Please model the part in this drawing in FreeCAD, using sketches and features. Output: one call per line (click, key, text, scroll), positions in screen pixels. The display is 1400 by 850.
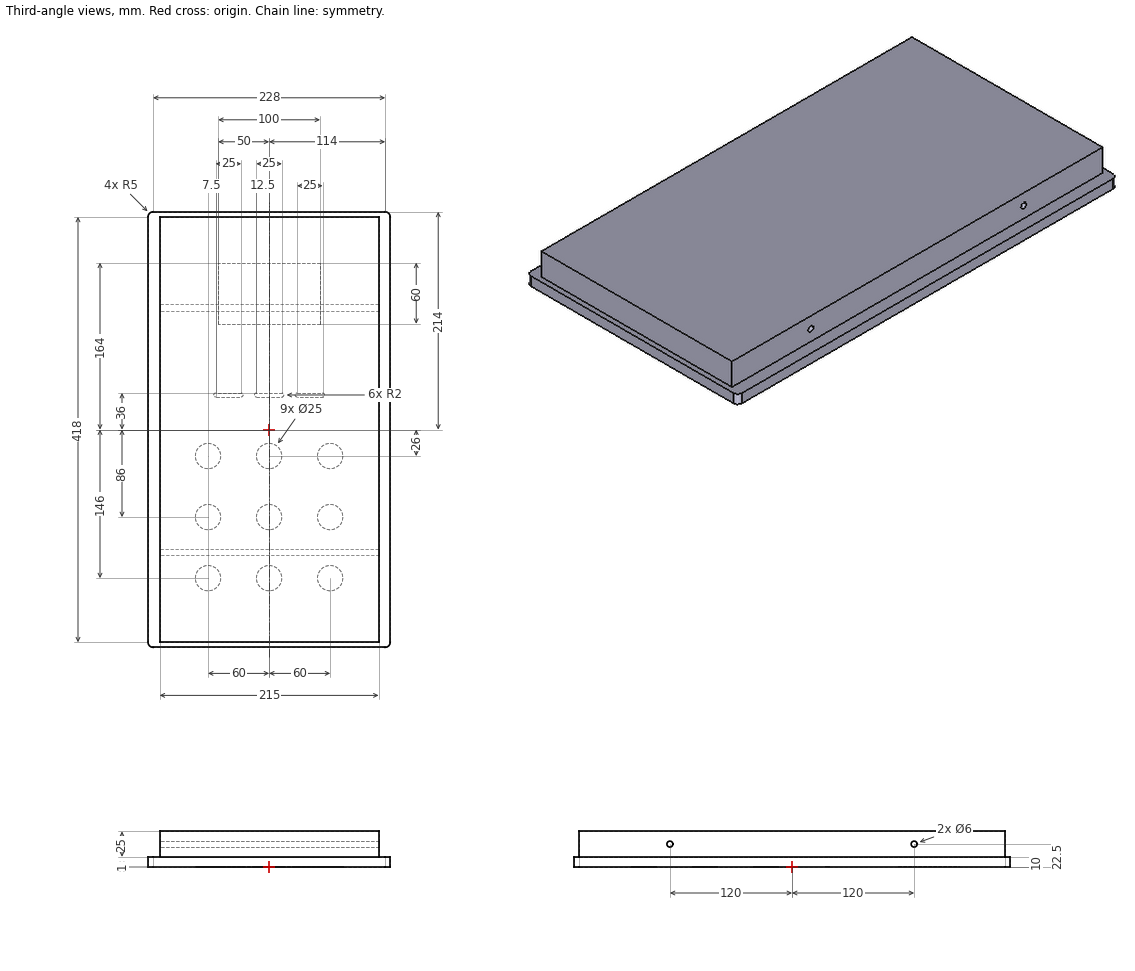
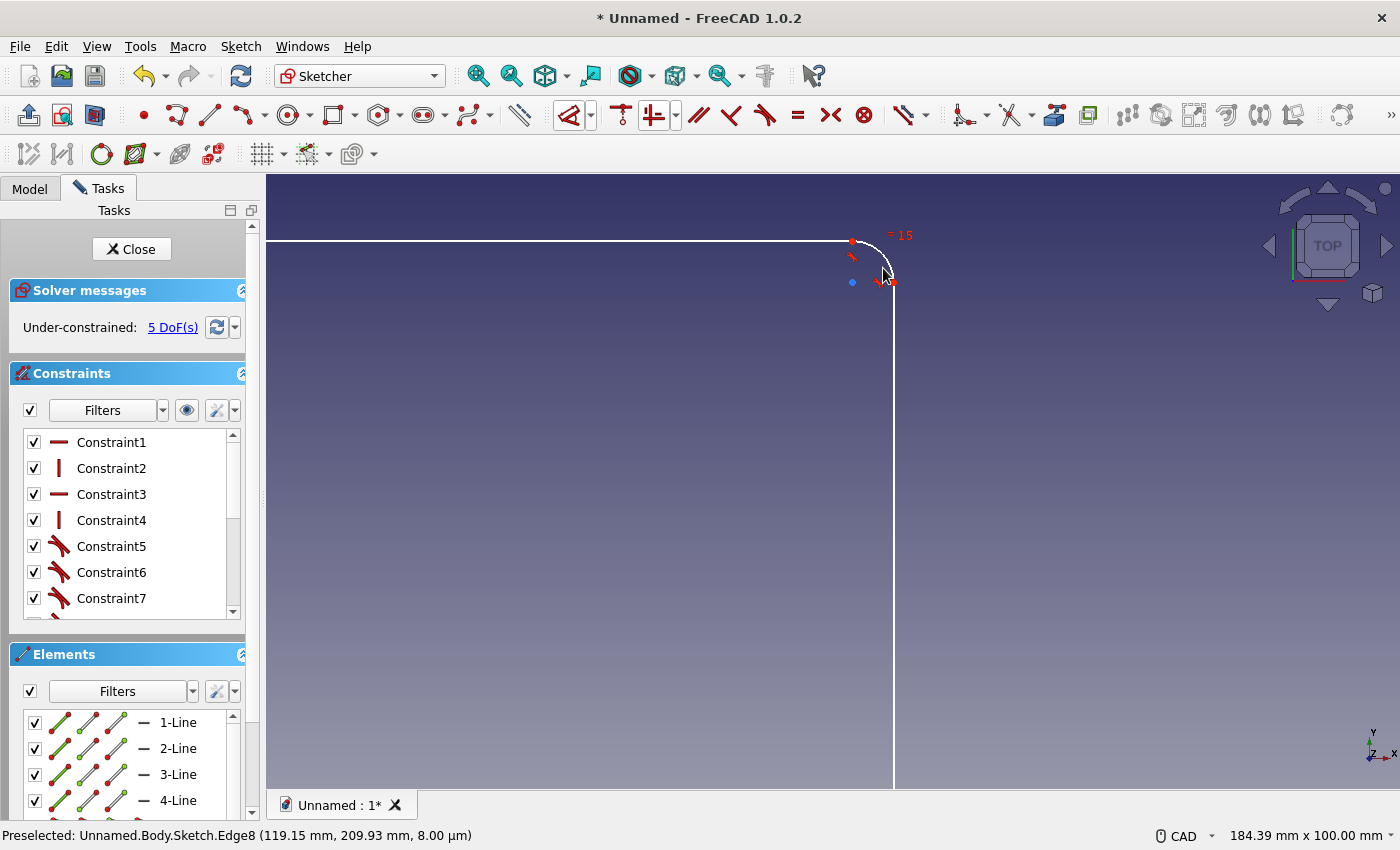
click(568, 116)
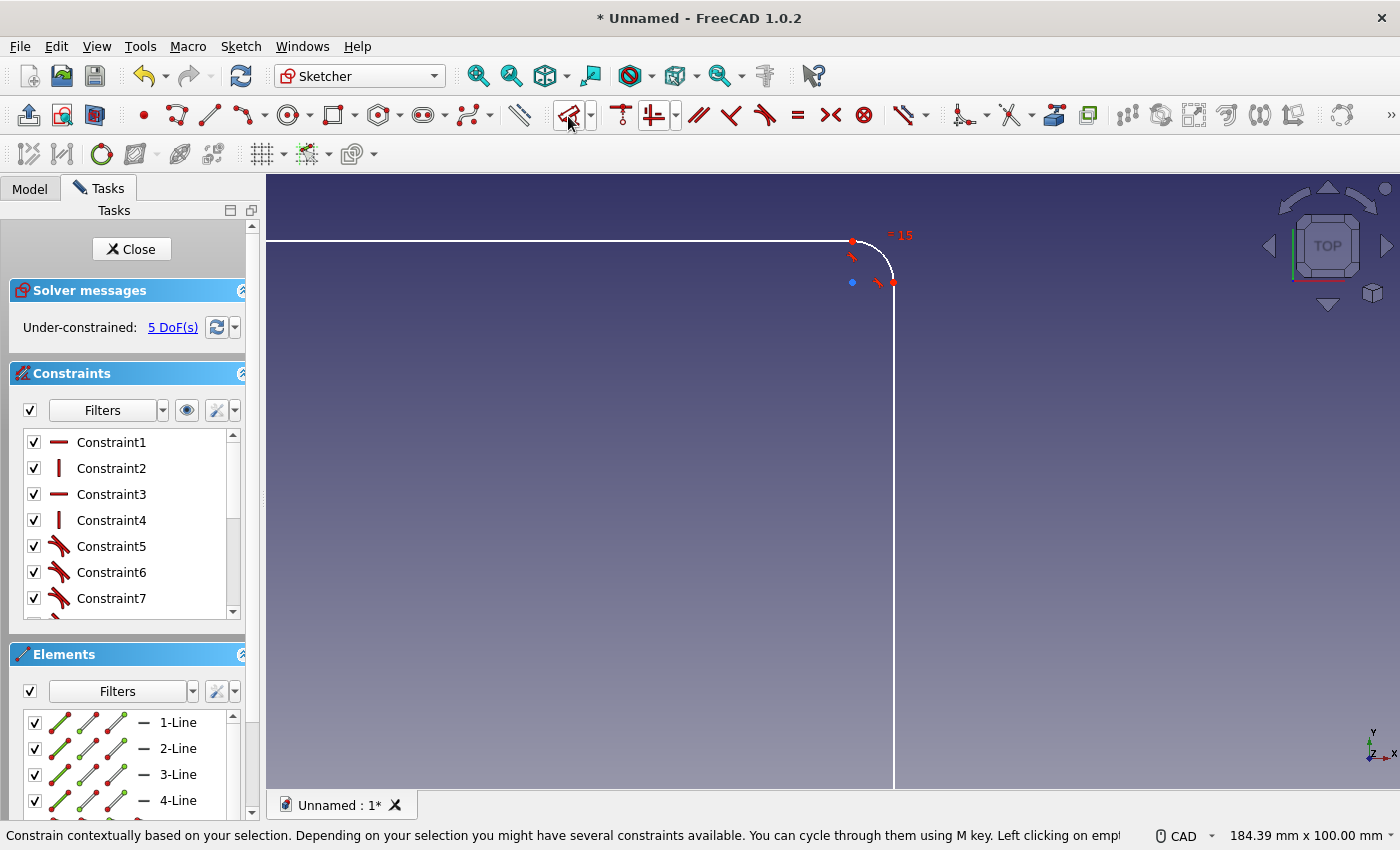
scroll(886, 267, down, 9)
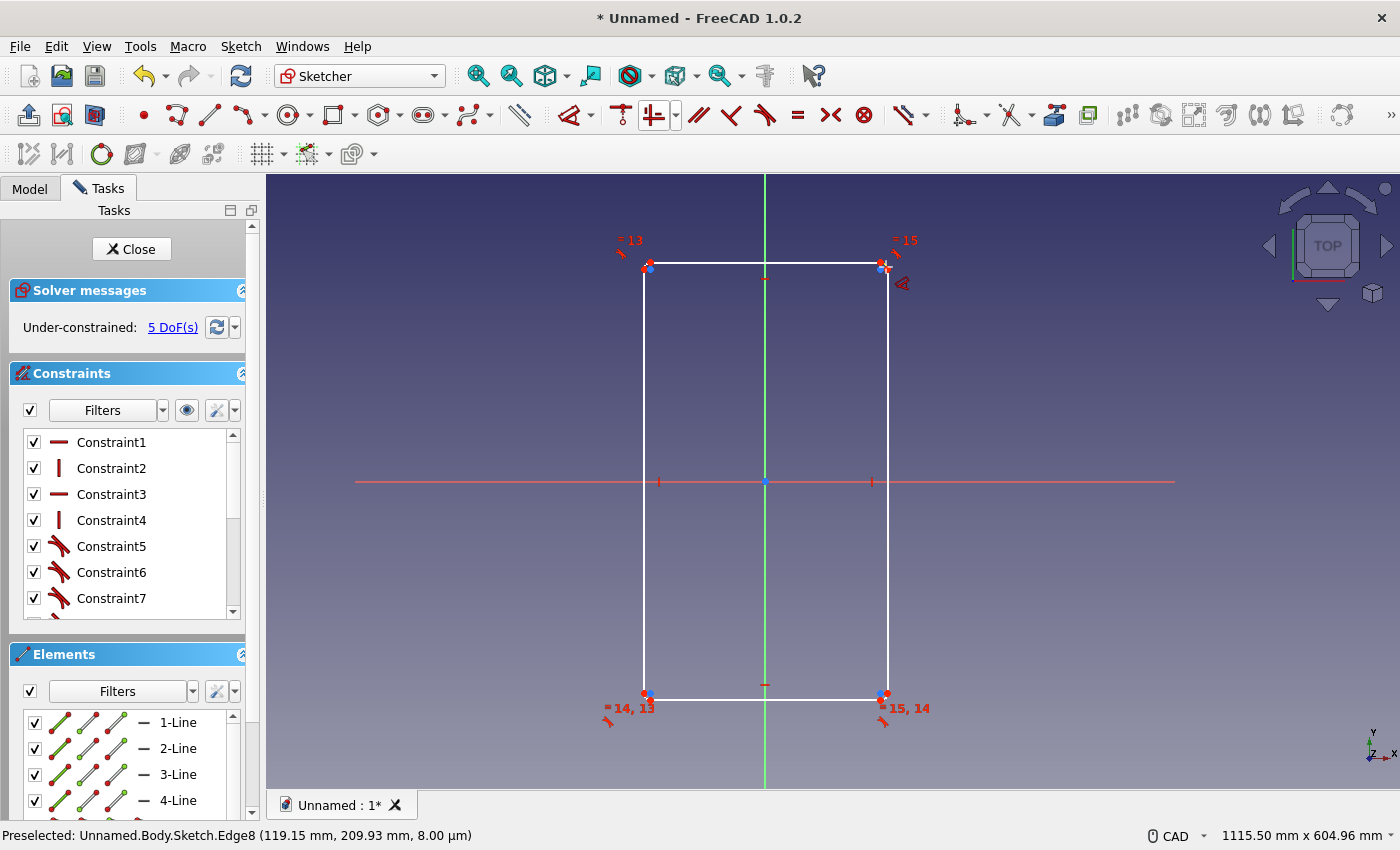
scroll(648, 264, up, 11)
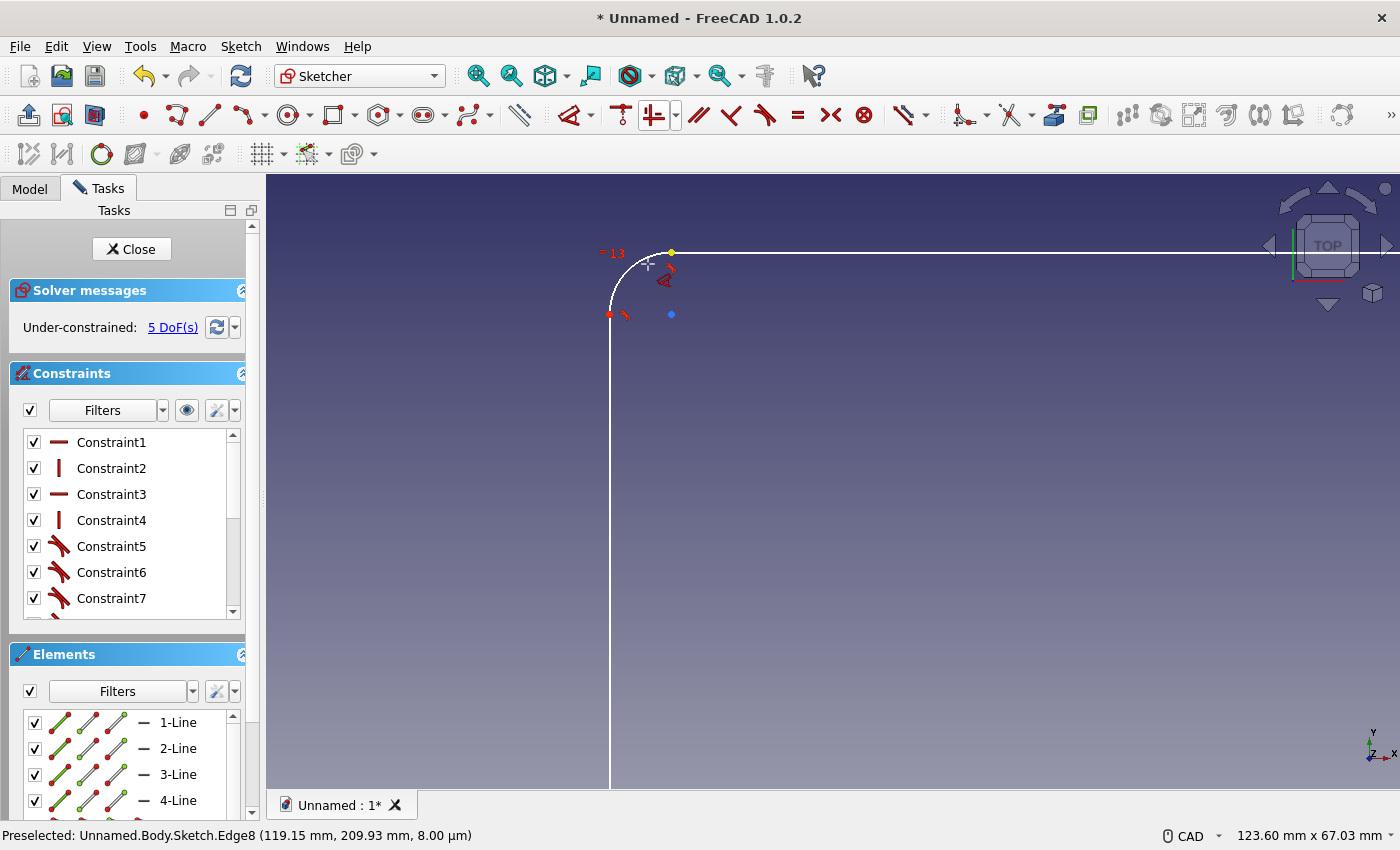
click(643, 259)
click(628, 231)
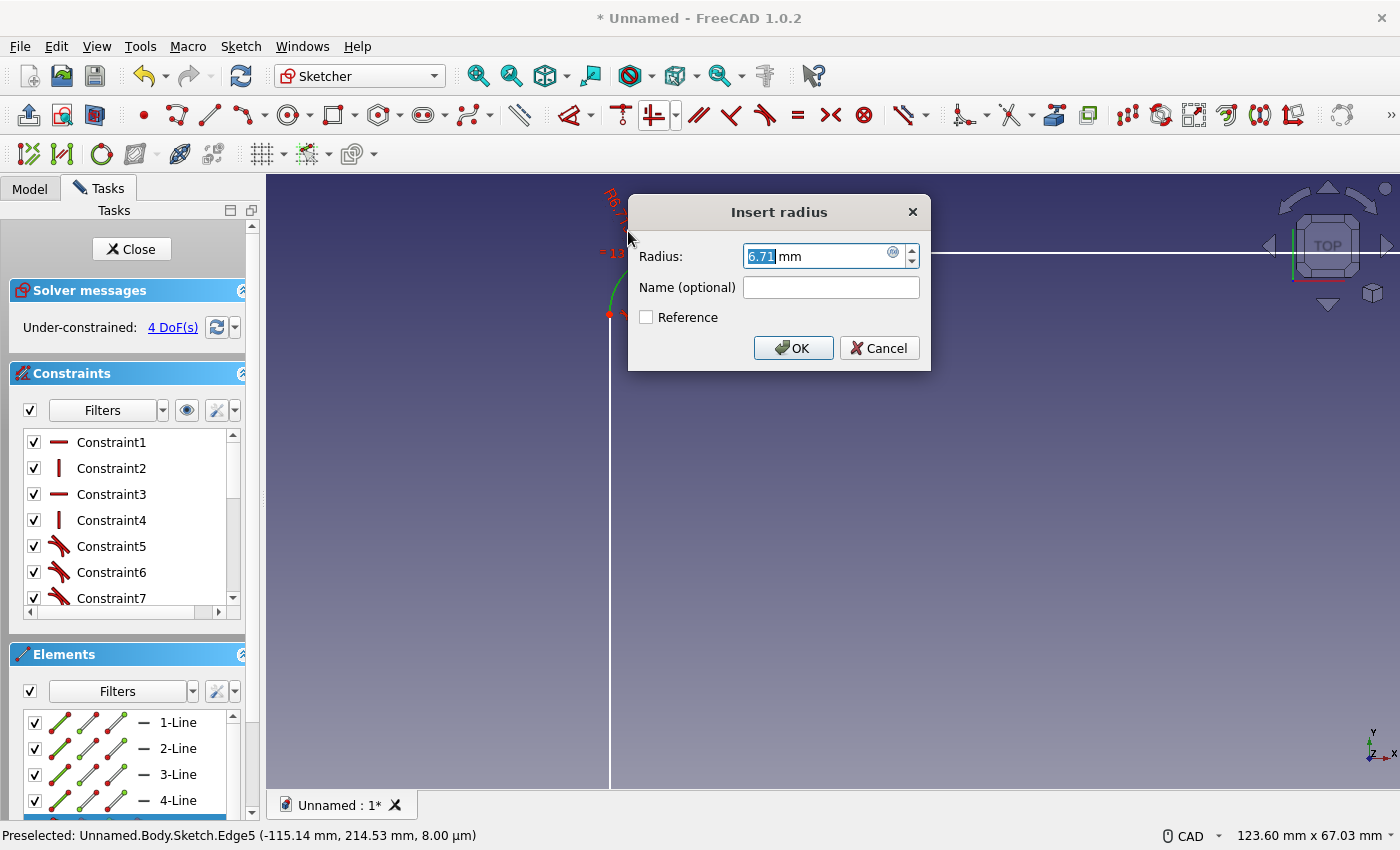
text(5)
key(Return)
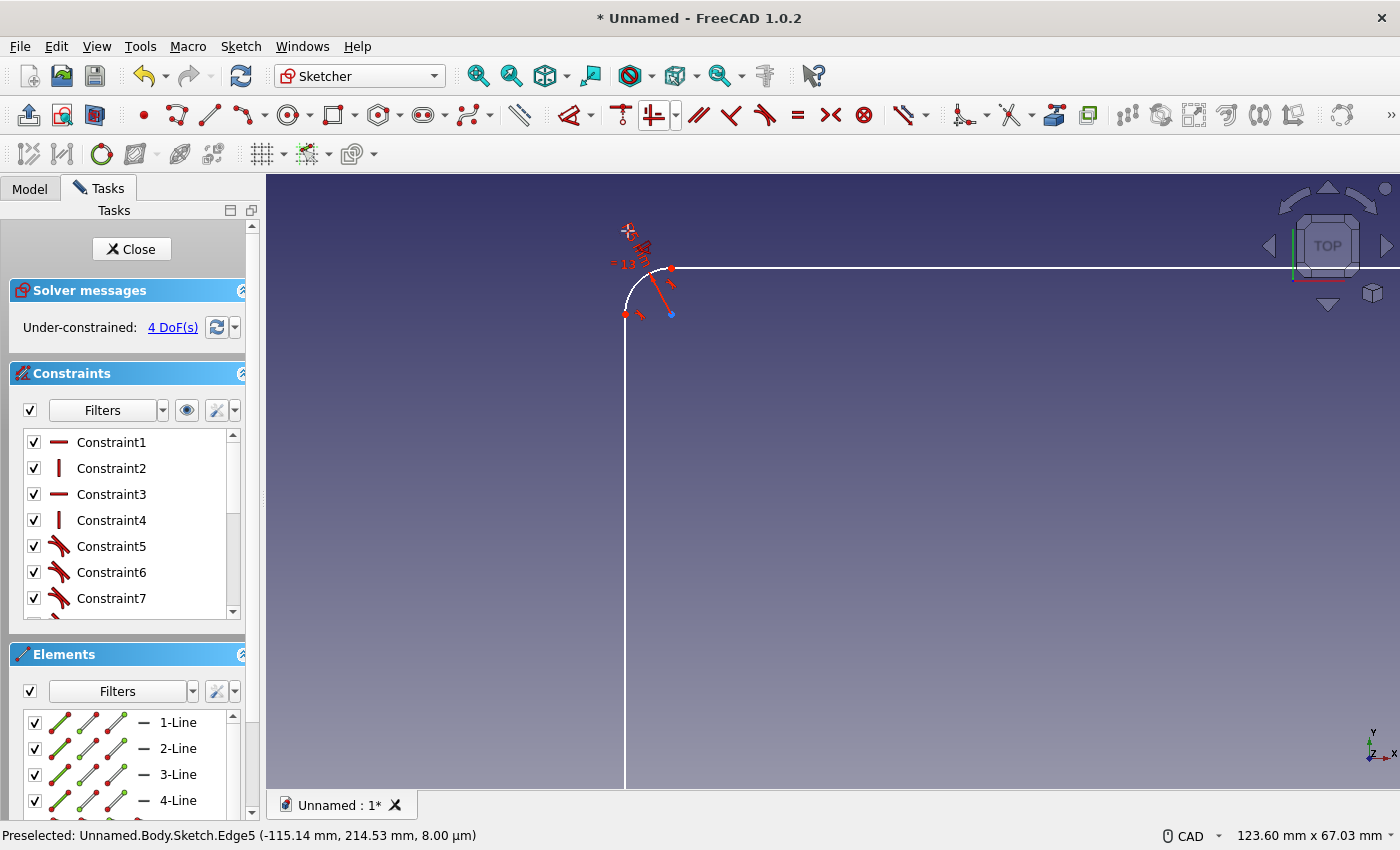
scroll(648, 264, down, 11)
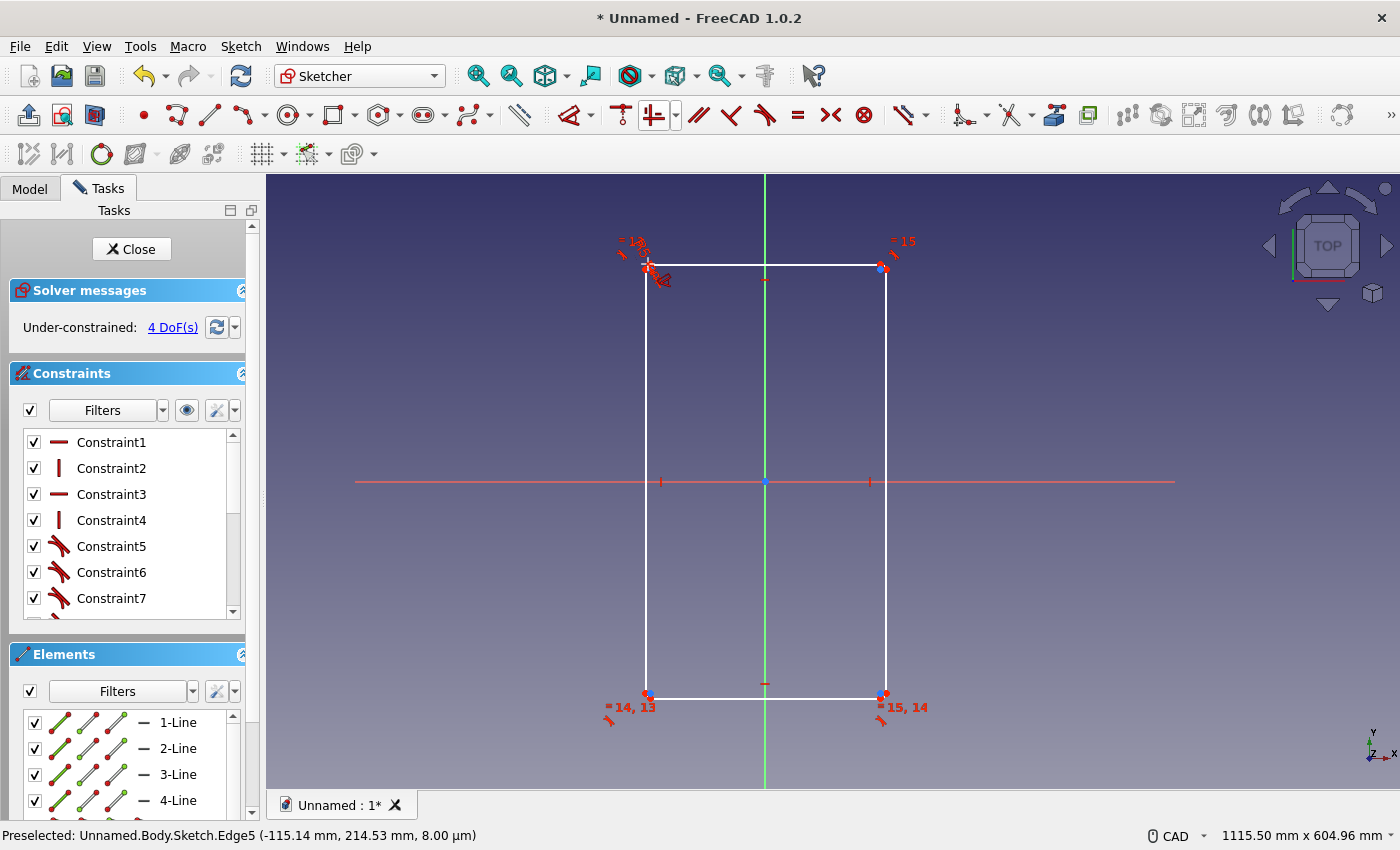
click(697, 265)
click(713, 231)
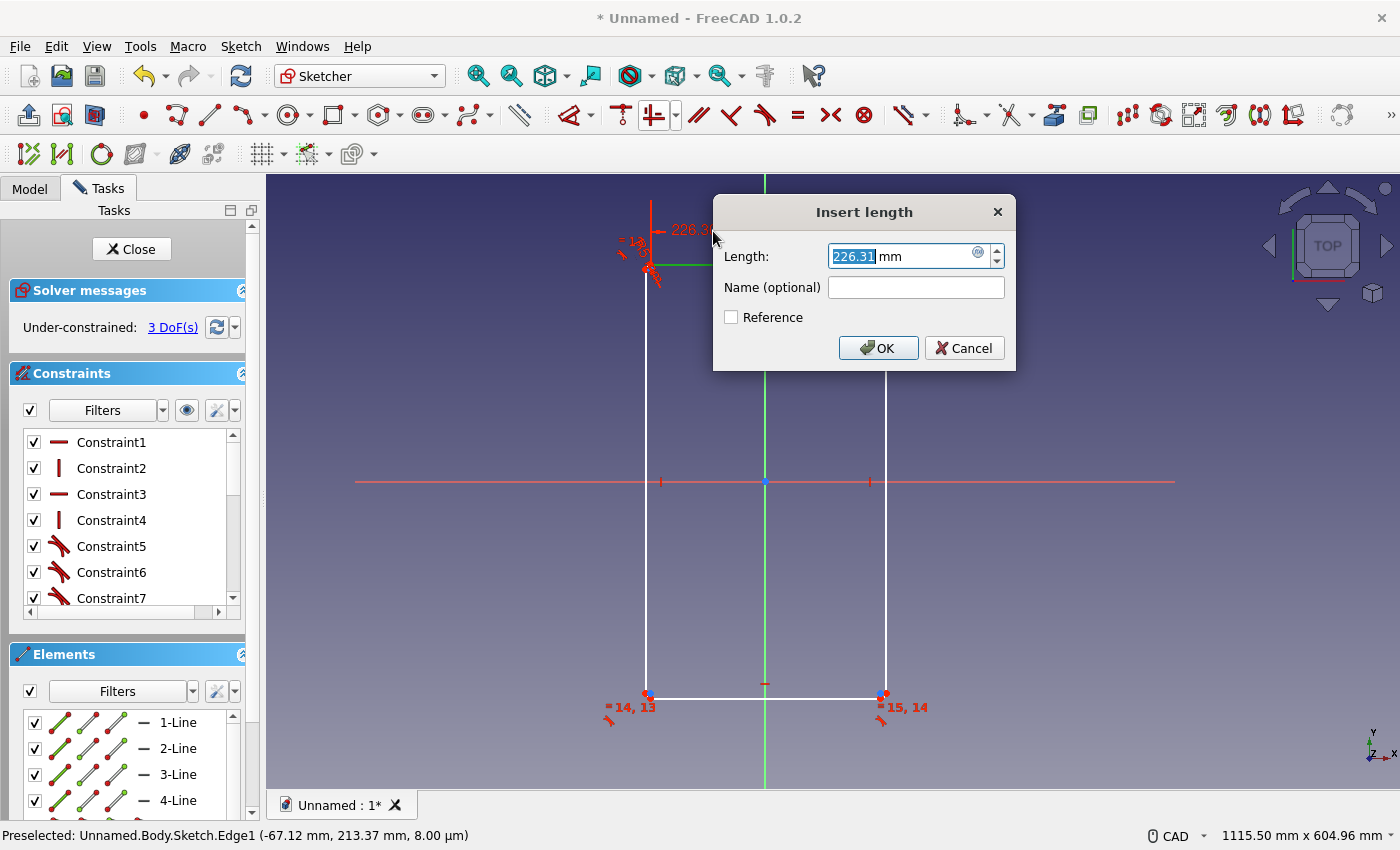
text(228)
key(Return)